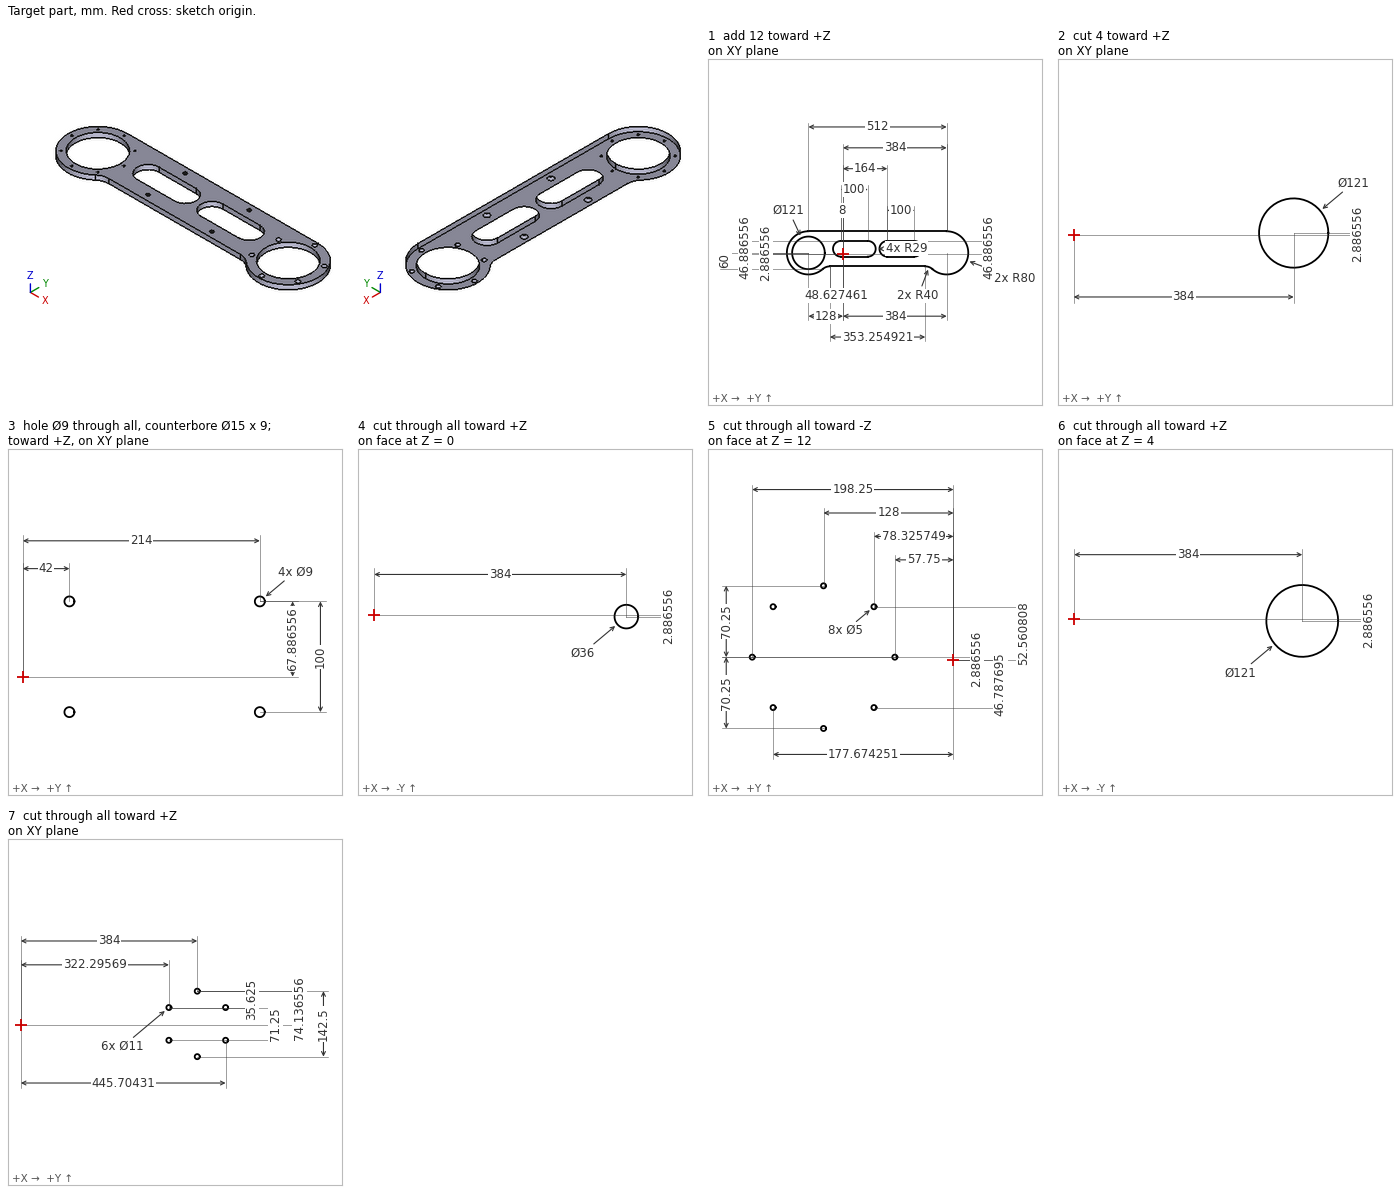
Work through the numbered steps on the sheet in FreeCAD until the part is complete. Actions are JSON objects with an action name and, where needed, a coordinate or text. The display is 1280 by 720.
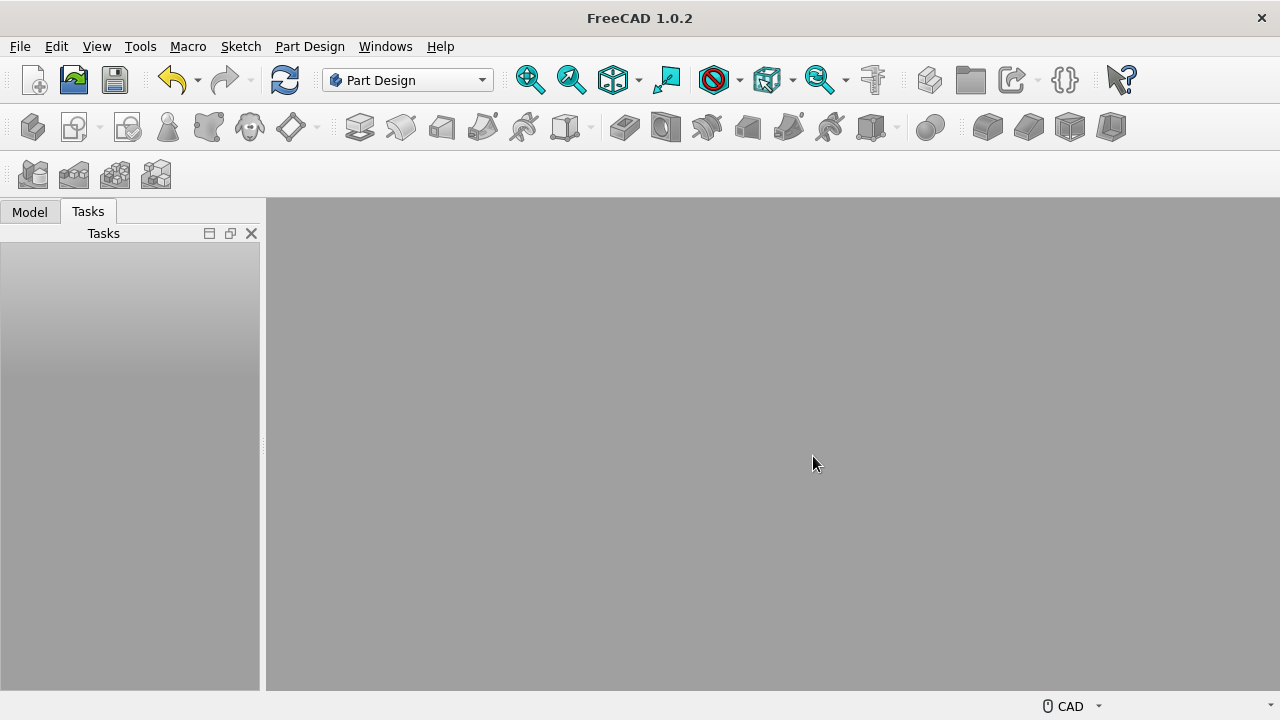
{"action": "left_click", "coordinate": [33, 80]}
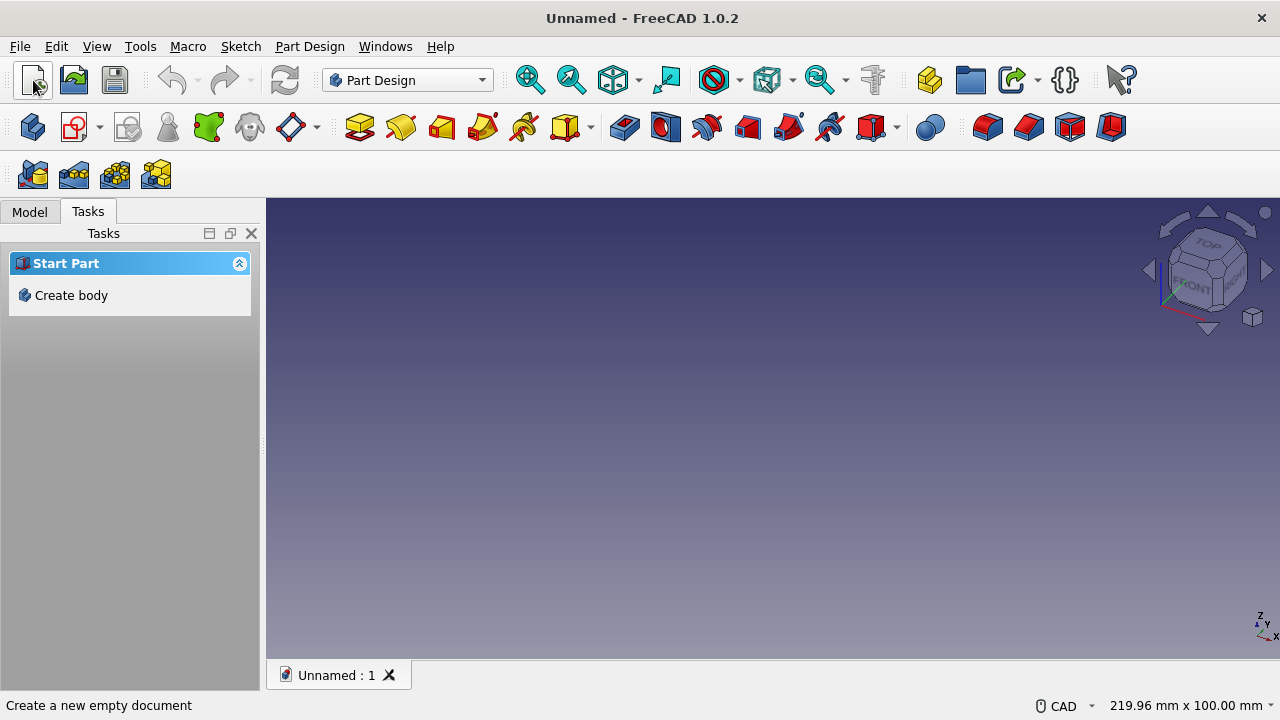
{"action": "left_click", "coordinate": [74, 128]}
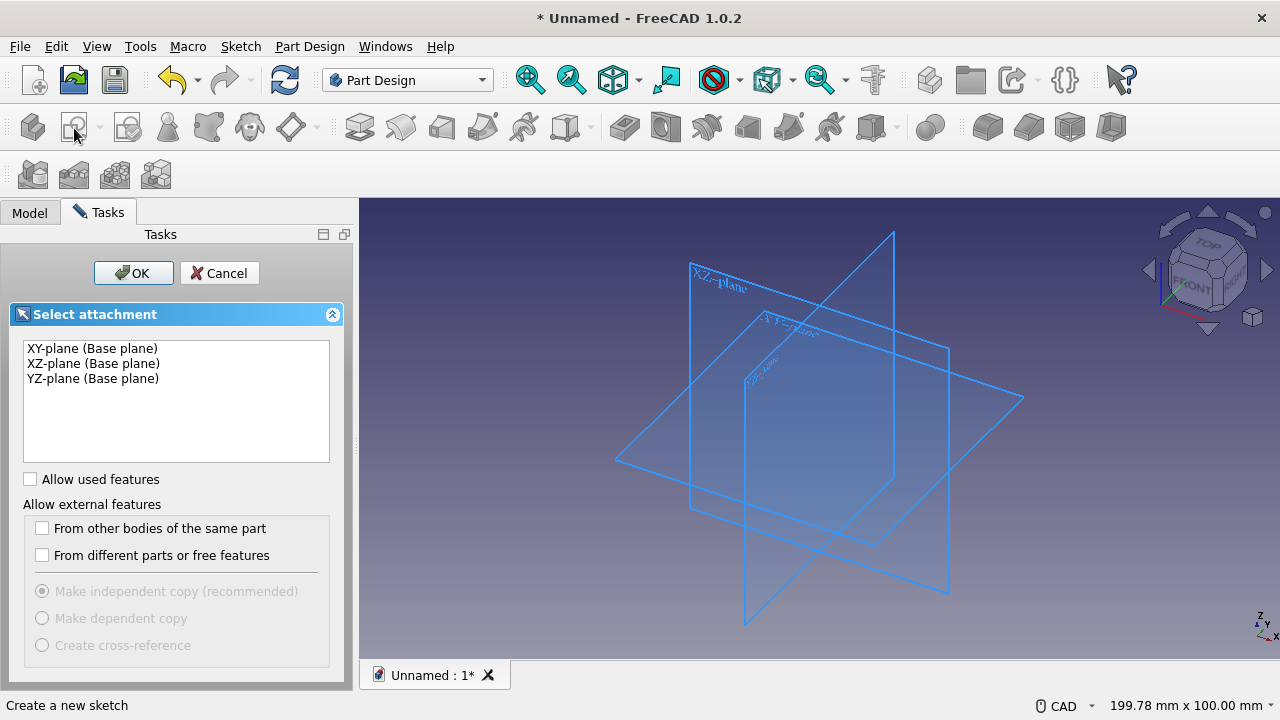
{"action": "left_click", "coordinate": [84, 348]}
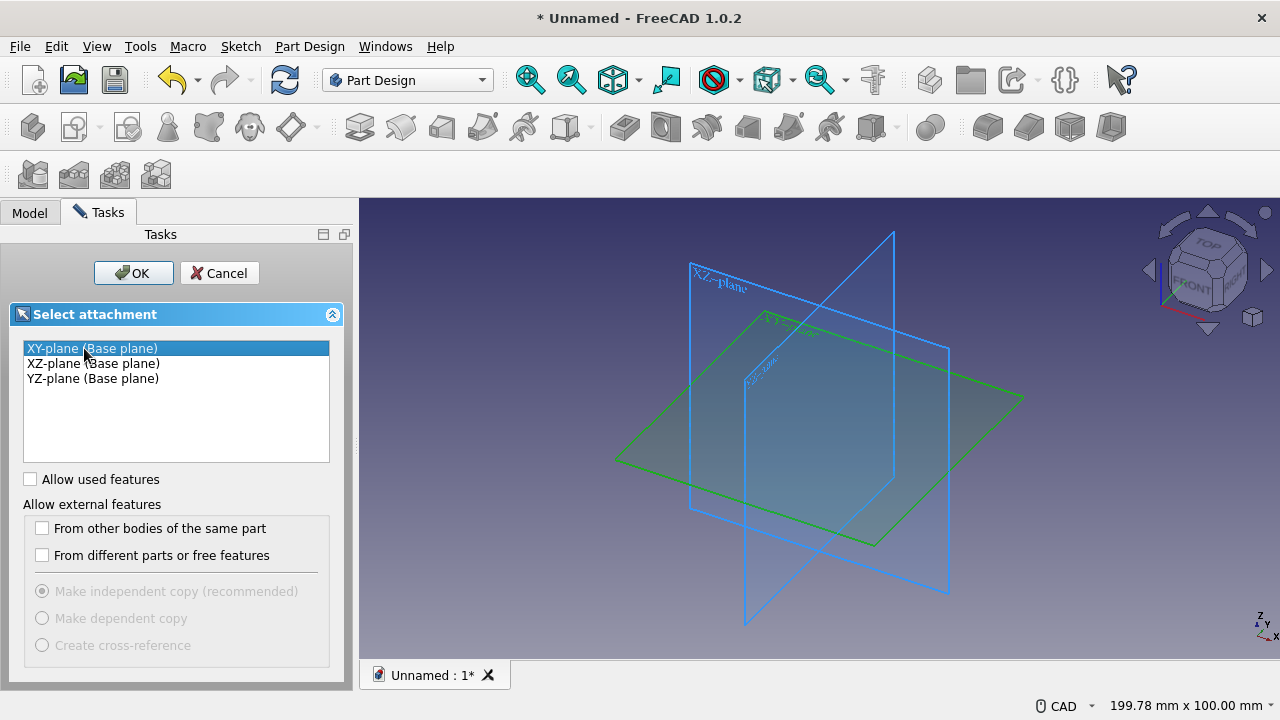
{"action": "left_click", "coordinate": [134, 273]}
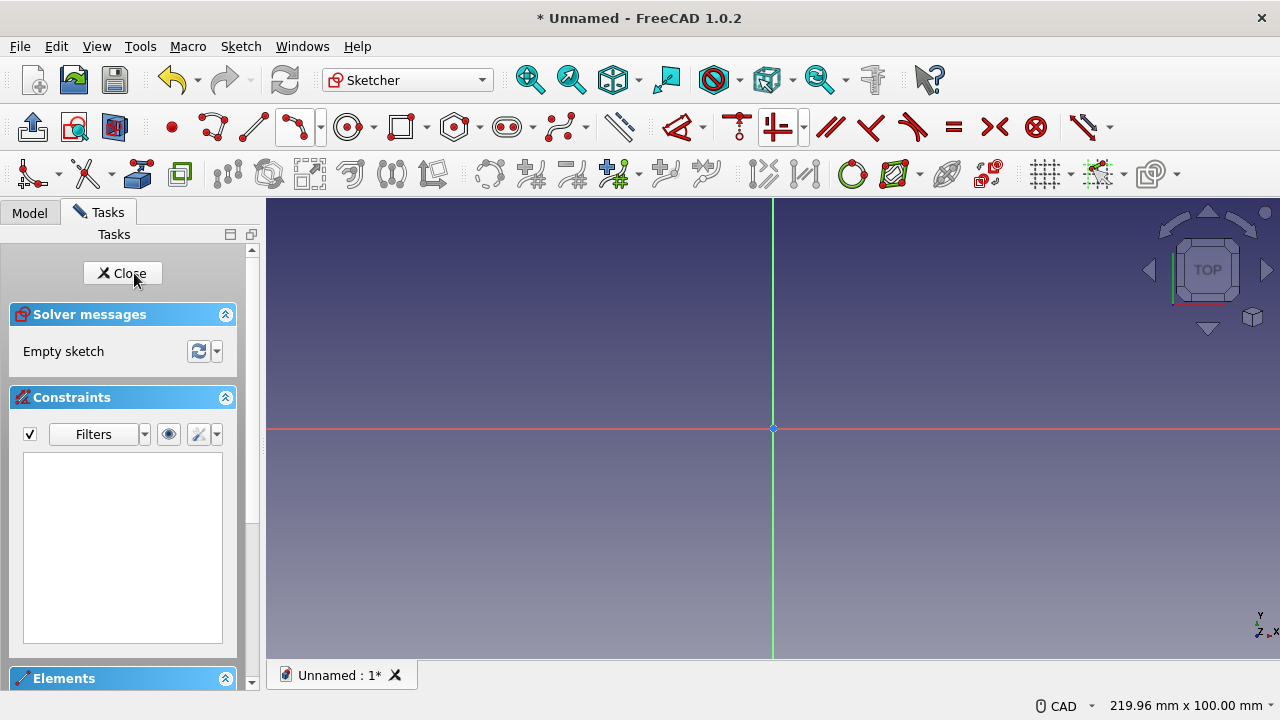
{"action": "scroll", "coordinate": [538, 443], "scroll_direction": "down", "scroll_amount": 8}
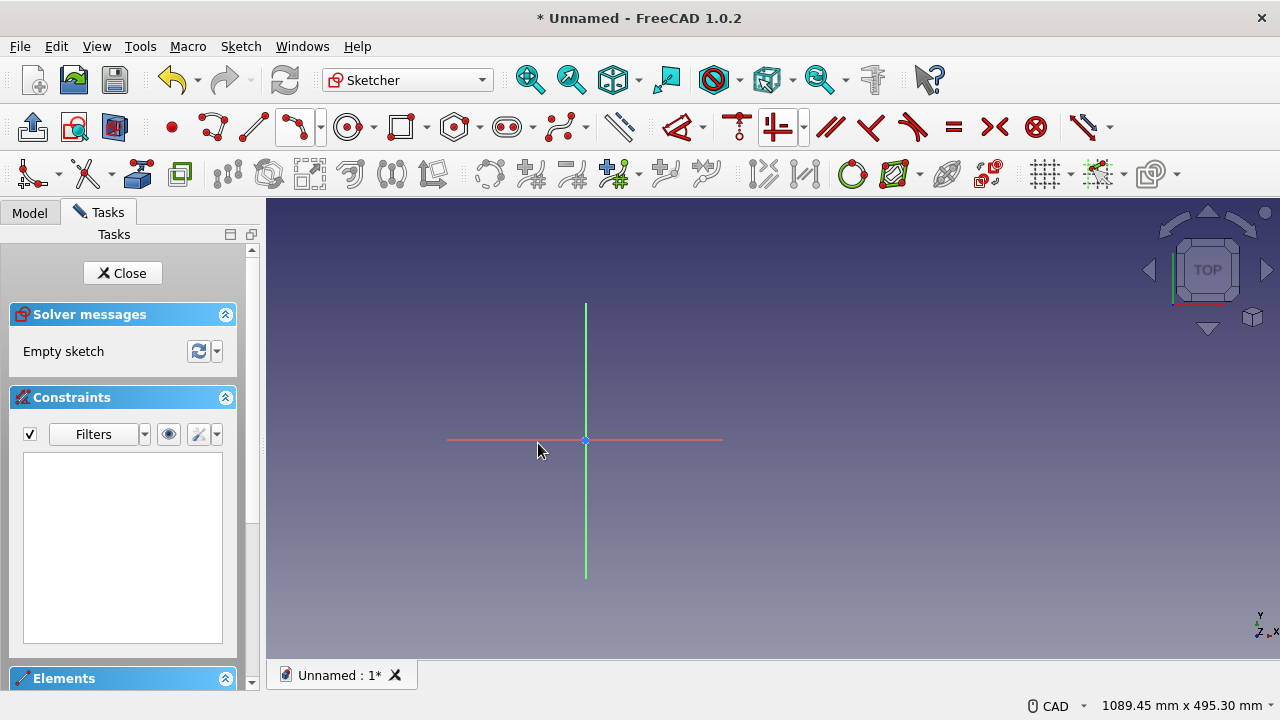
{"action": "left_click", "coordinate": [254, 128]}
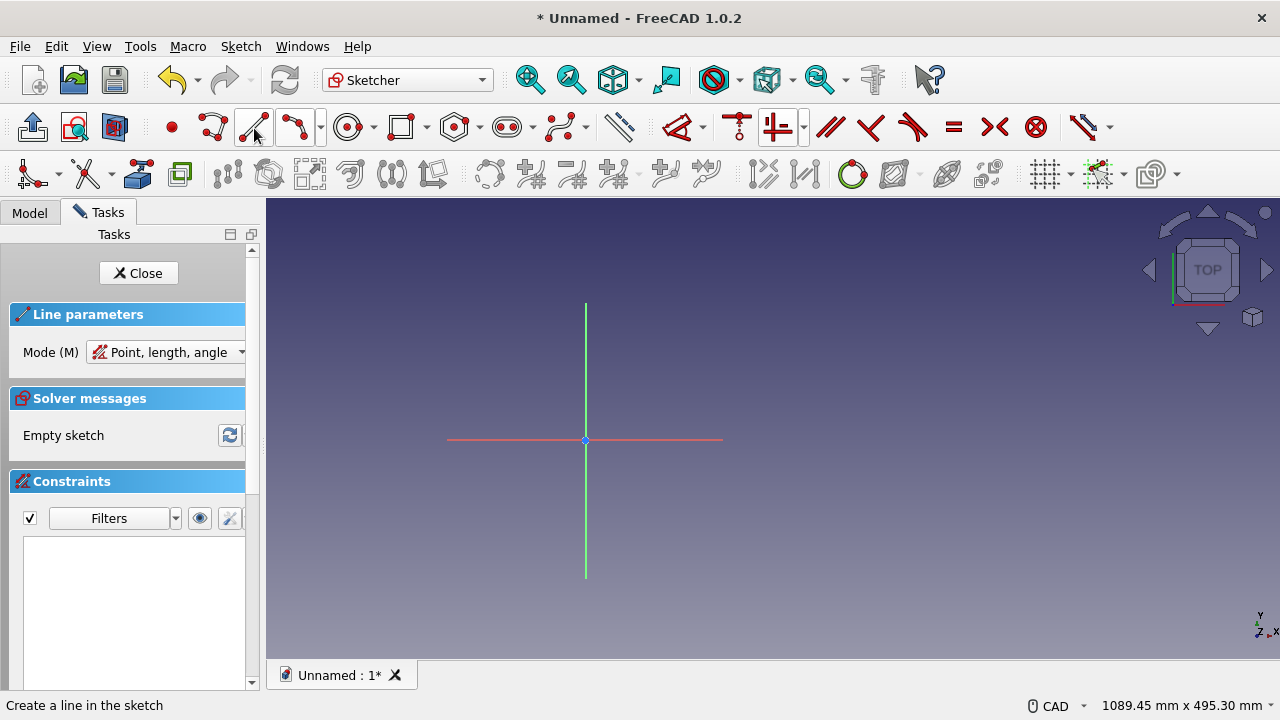
{"action": "left_click", "coordinate": [943, 363]}
{"action": "left_click", "coordinate": [467, 363]}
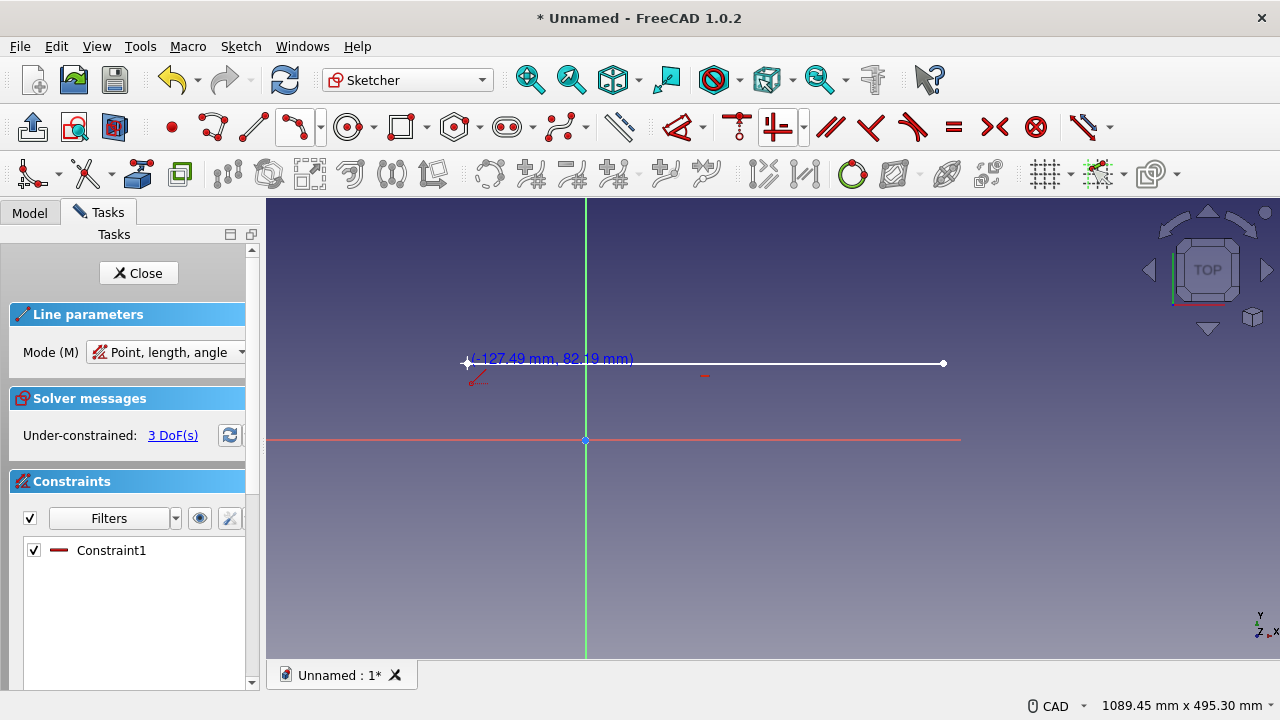
{"action": "left_click", "coordinate": [540, 484]}
{"action": "left_click", "coordinate": [869, 484]}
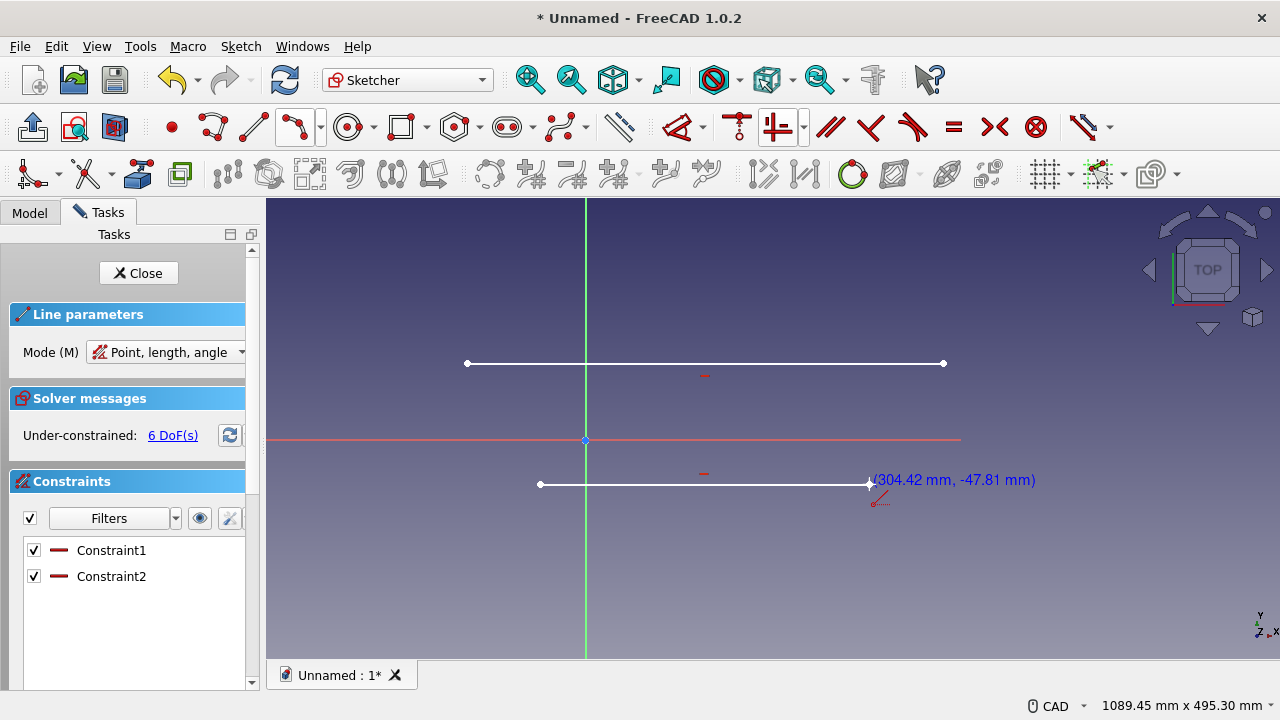
{"action": "left_click", "coordinate": [294, 128]}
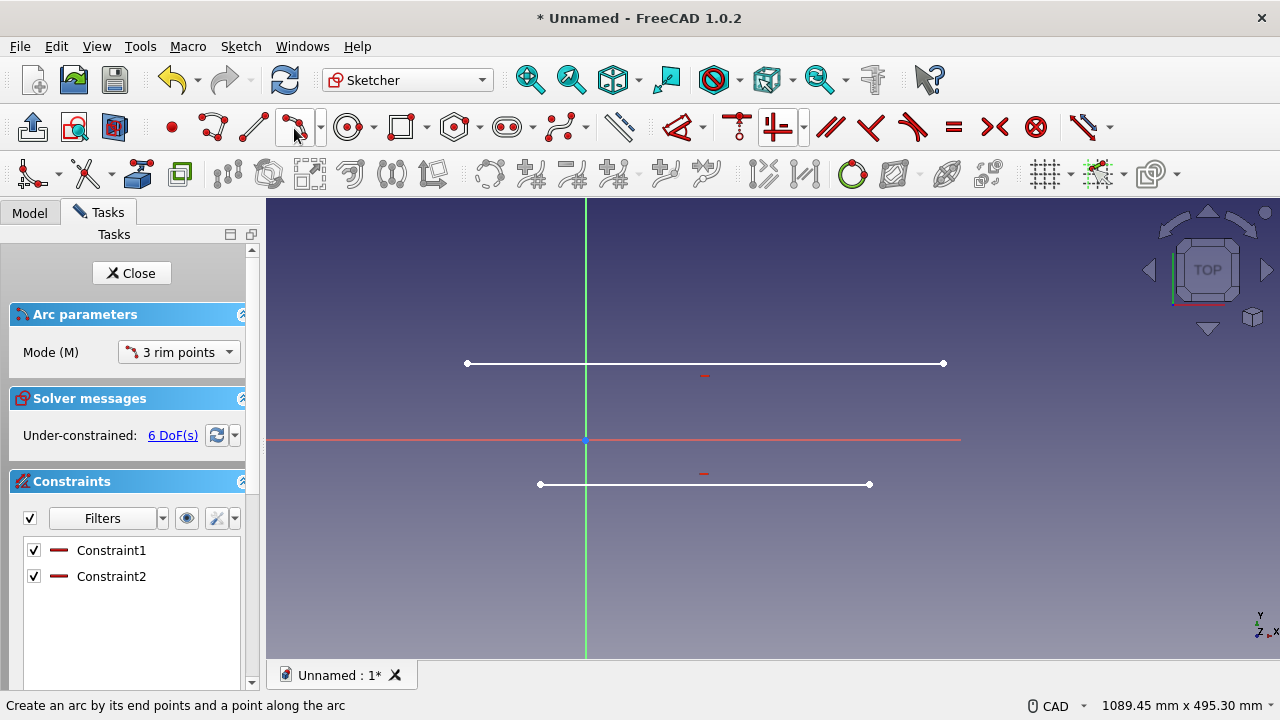
{"action": "left_click", "coordinate": [467, 364]}
{"action": "left_click", "coordinate": [516, 494]}
{"action": "left_click", "coordinate": [397, 464]}